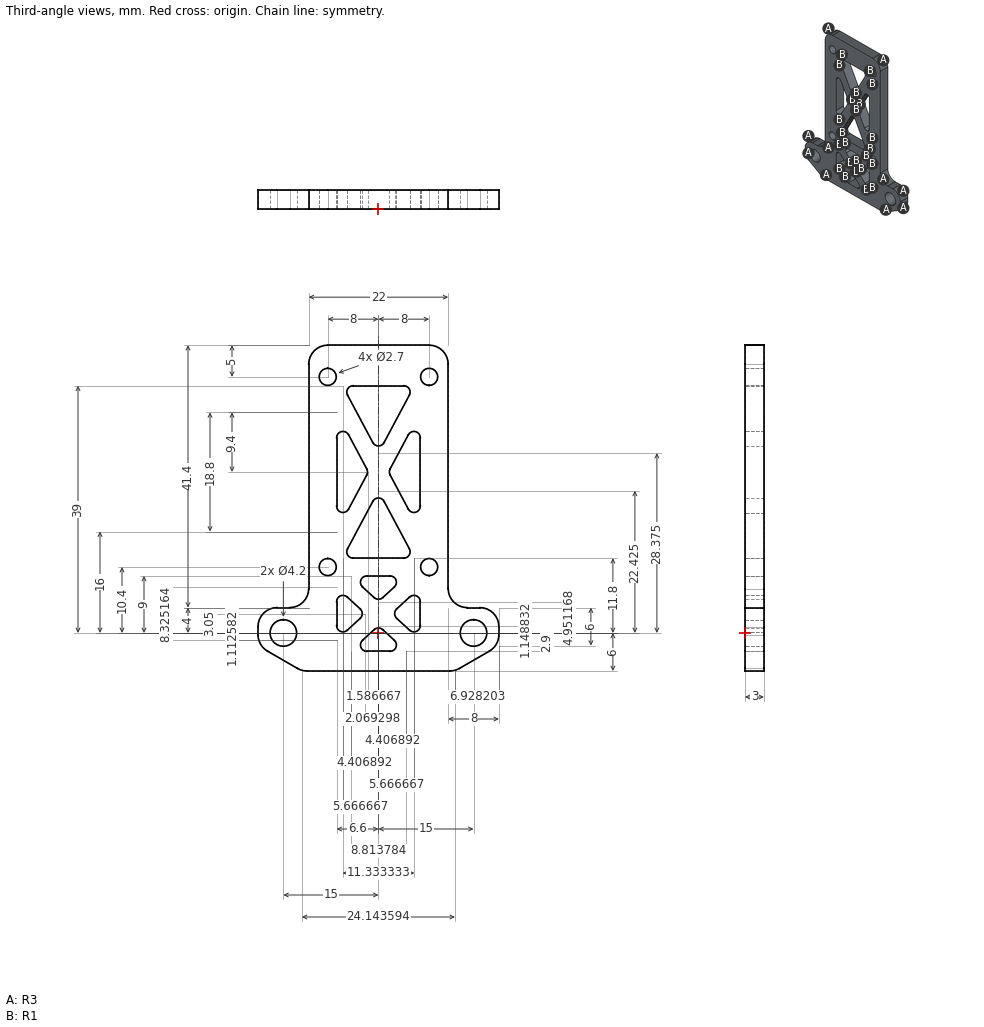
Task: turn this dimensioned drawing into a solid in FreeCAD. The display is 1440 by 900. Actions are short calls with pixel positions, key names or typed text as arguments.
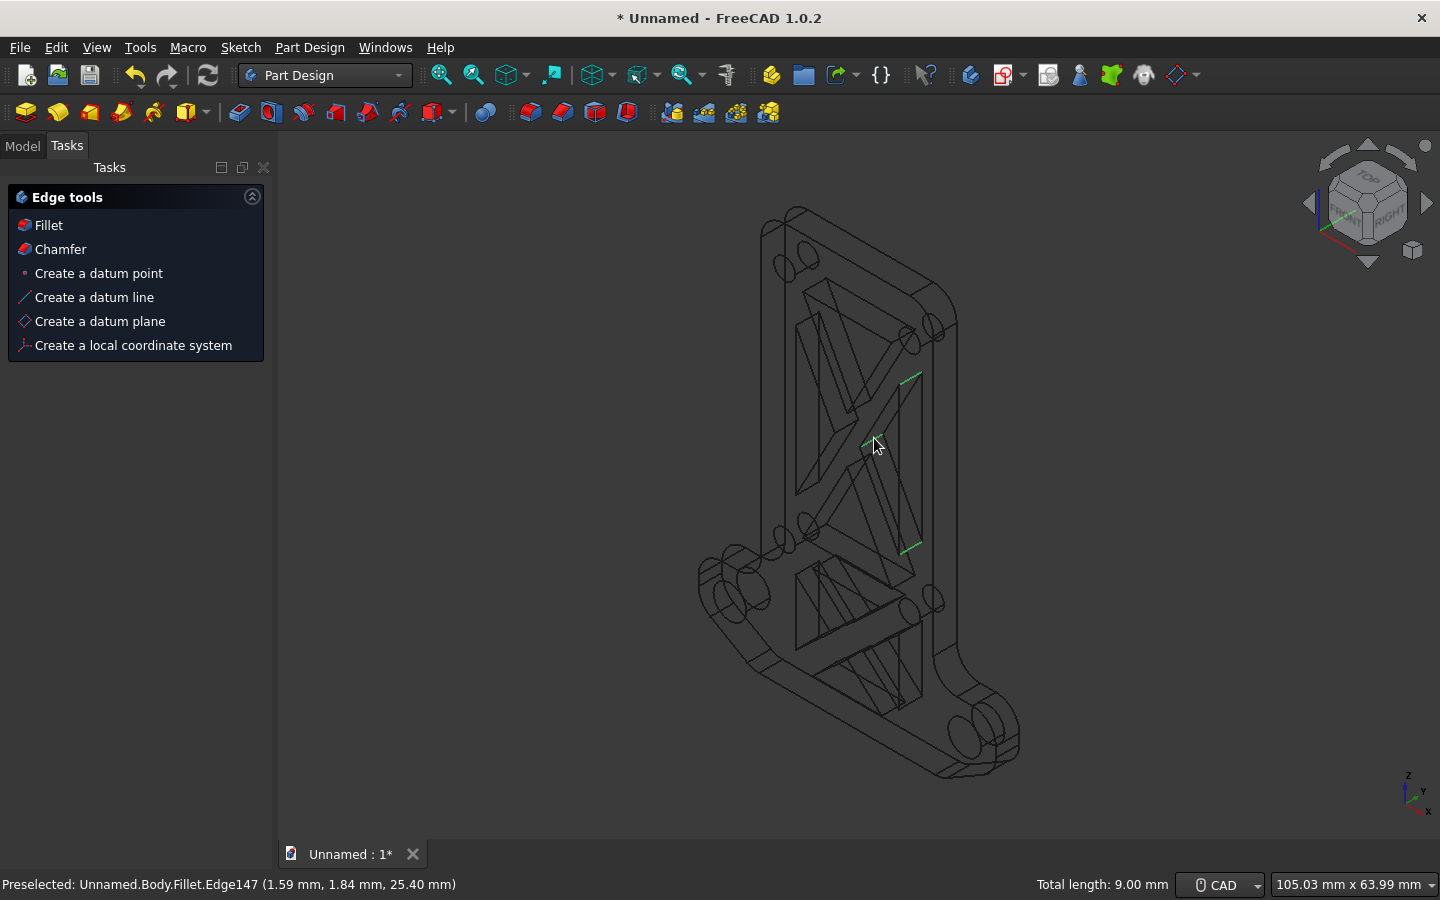
click(805, 319, ctrl)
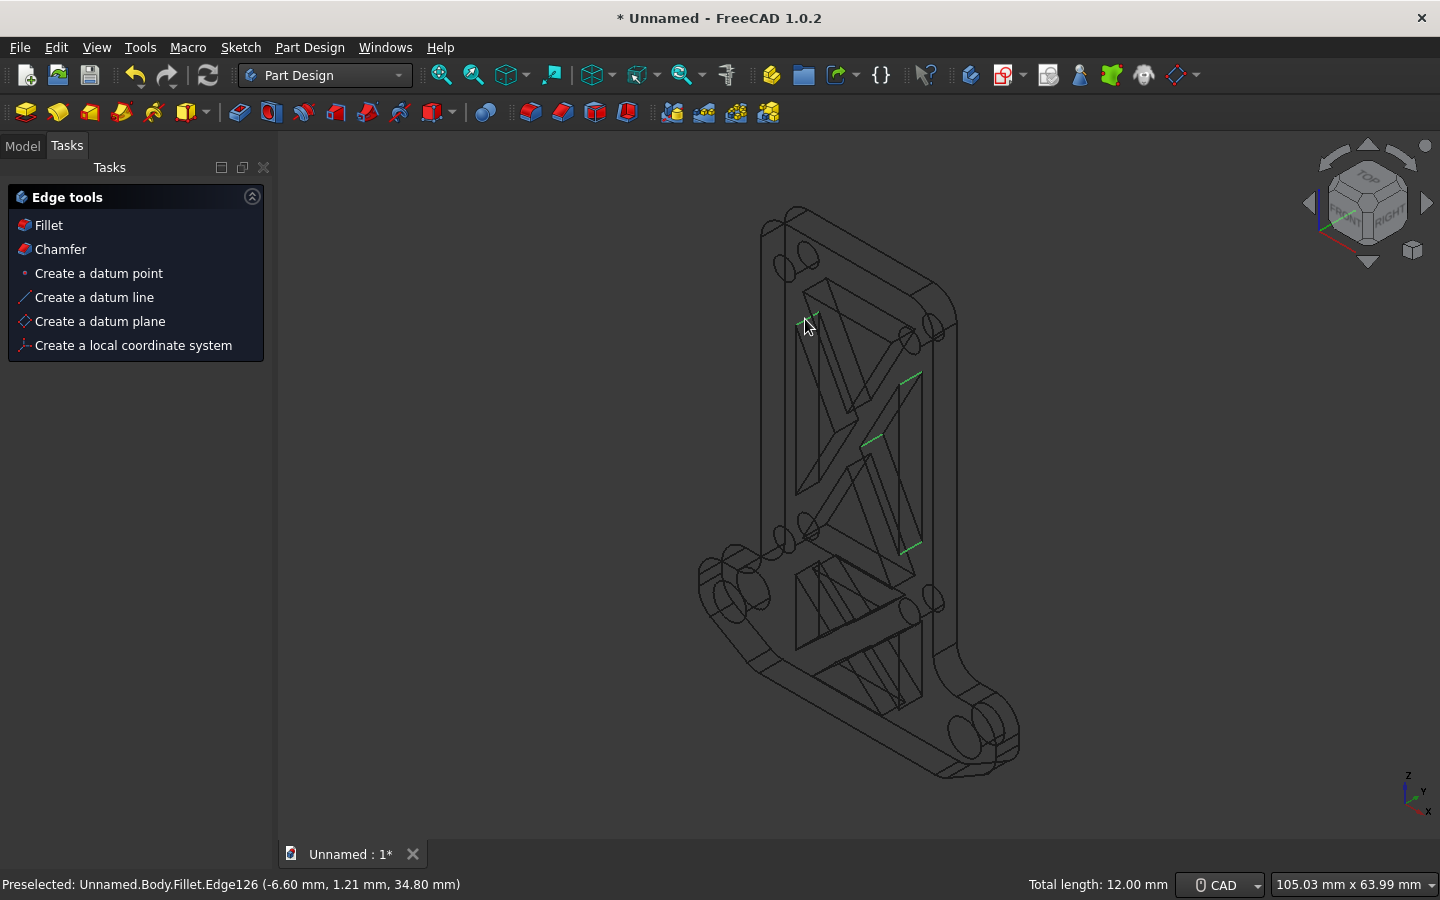
click(810, 486, ctrl)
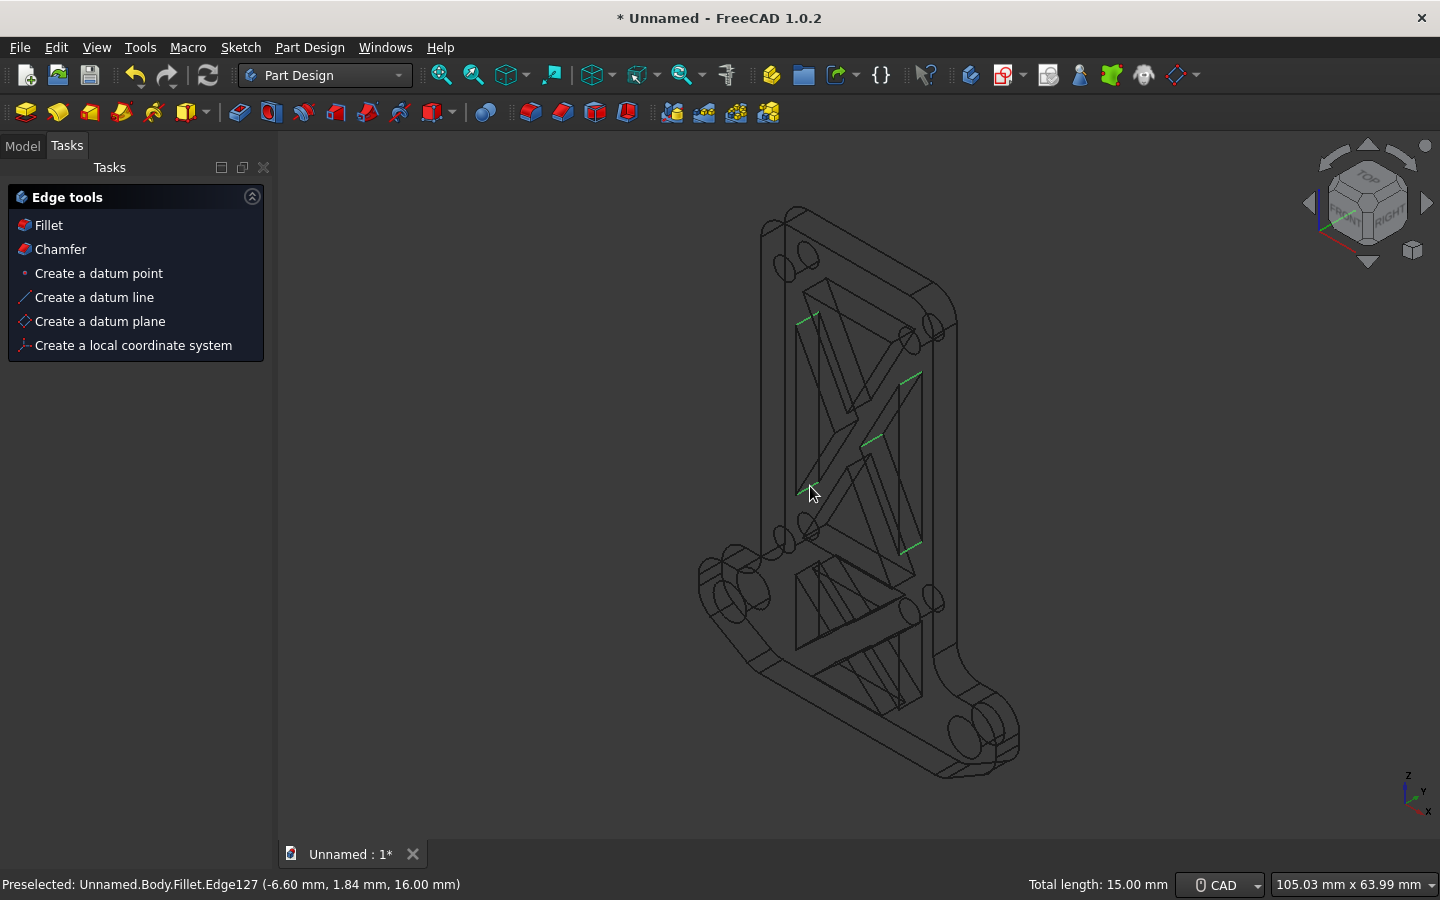
click(847, 425, ctrl)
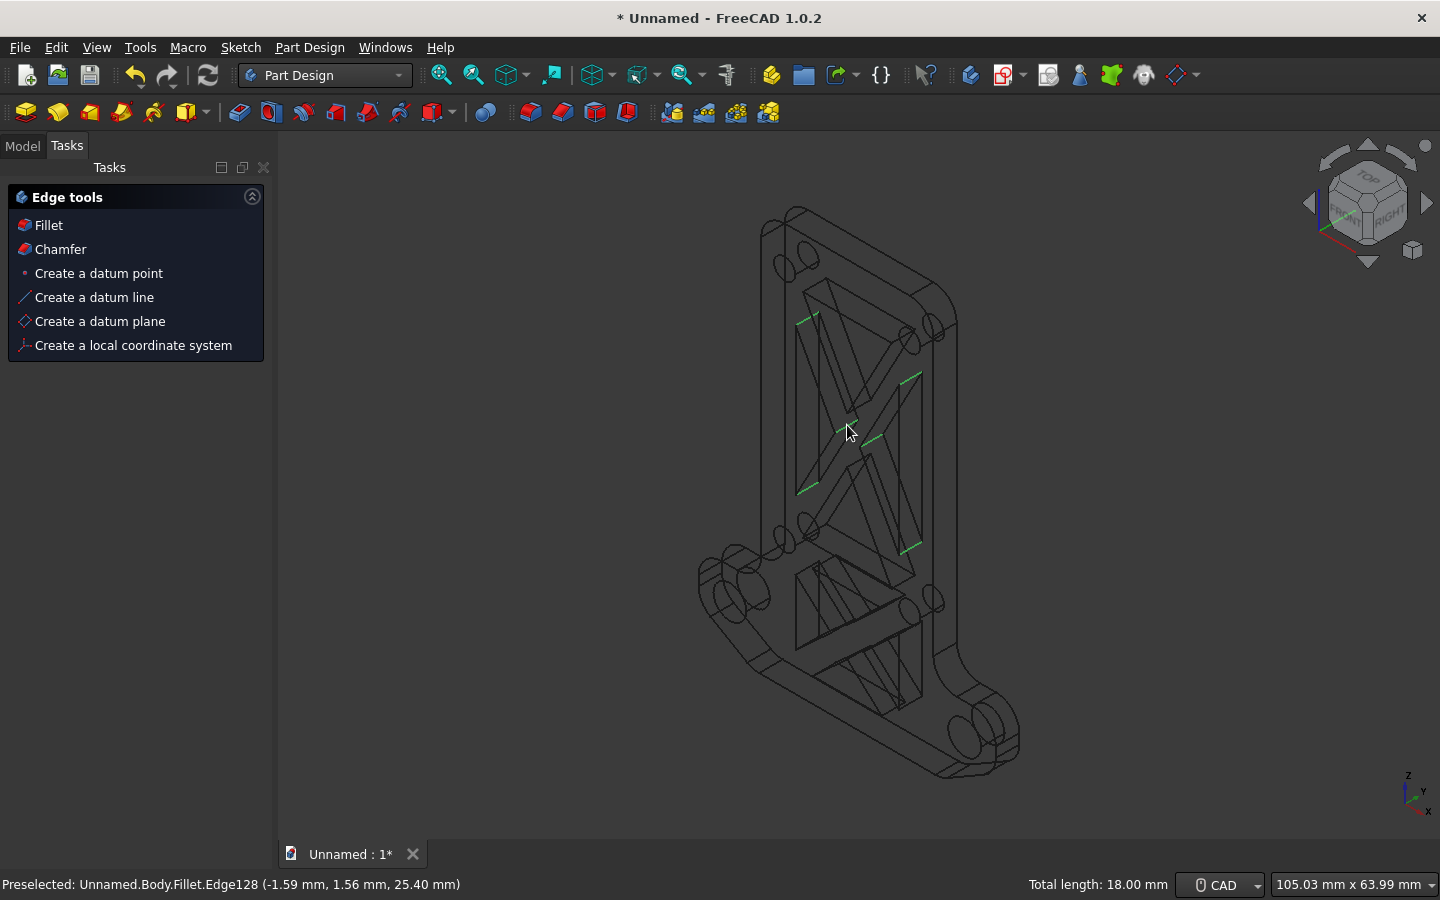
click(906, 334, ctrl)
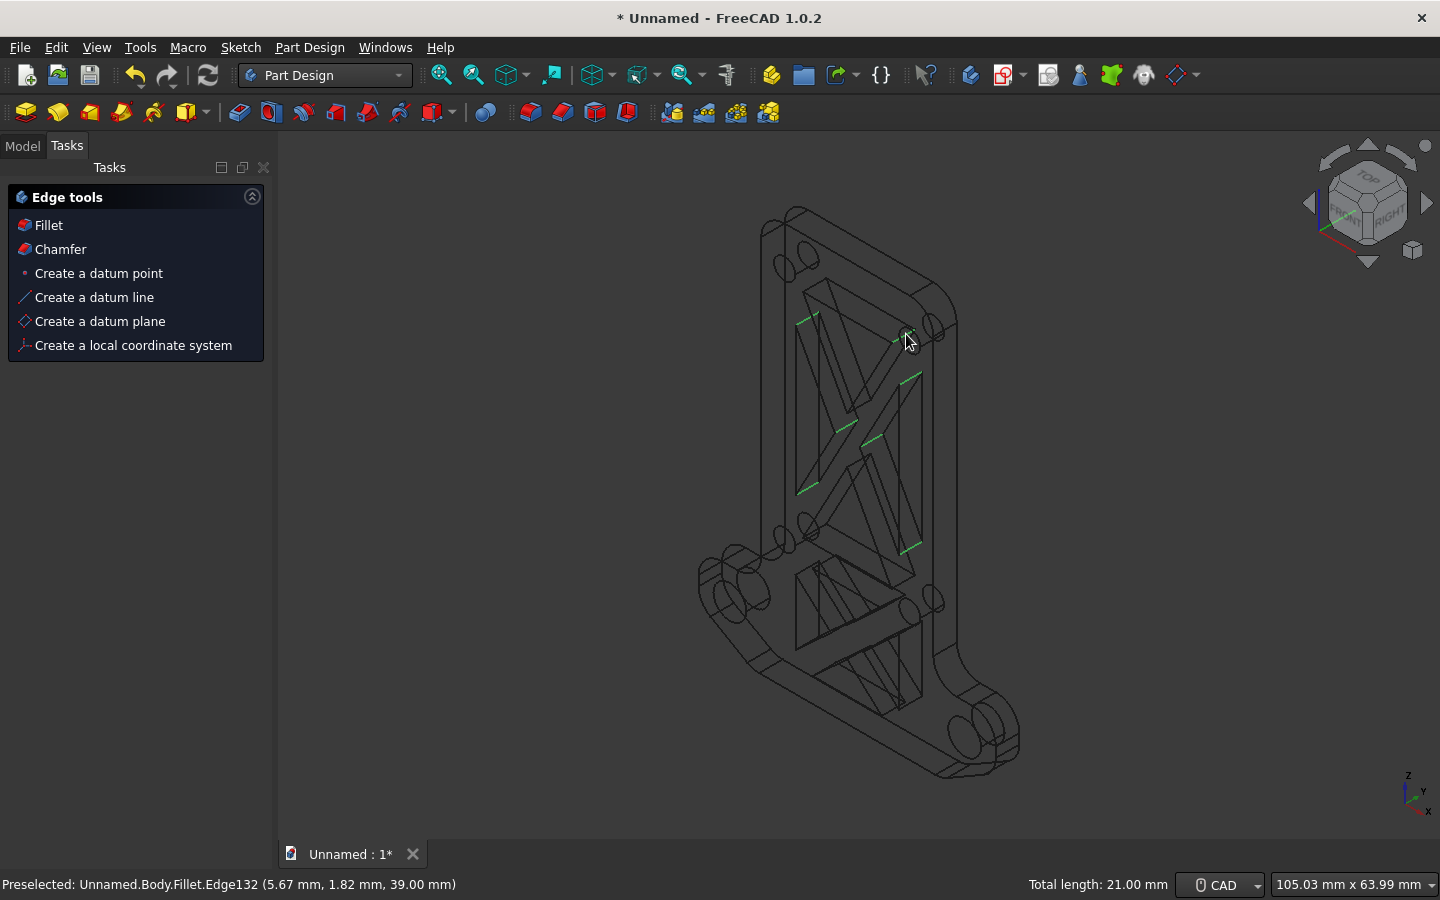
click(815, 284, ctrl)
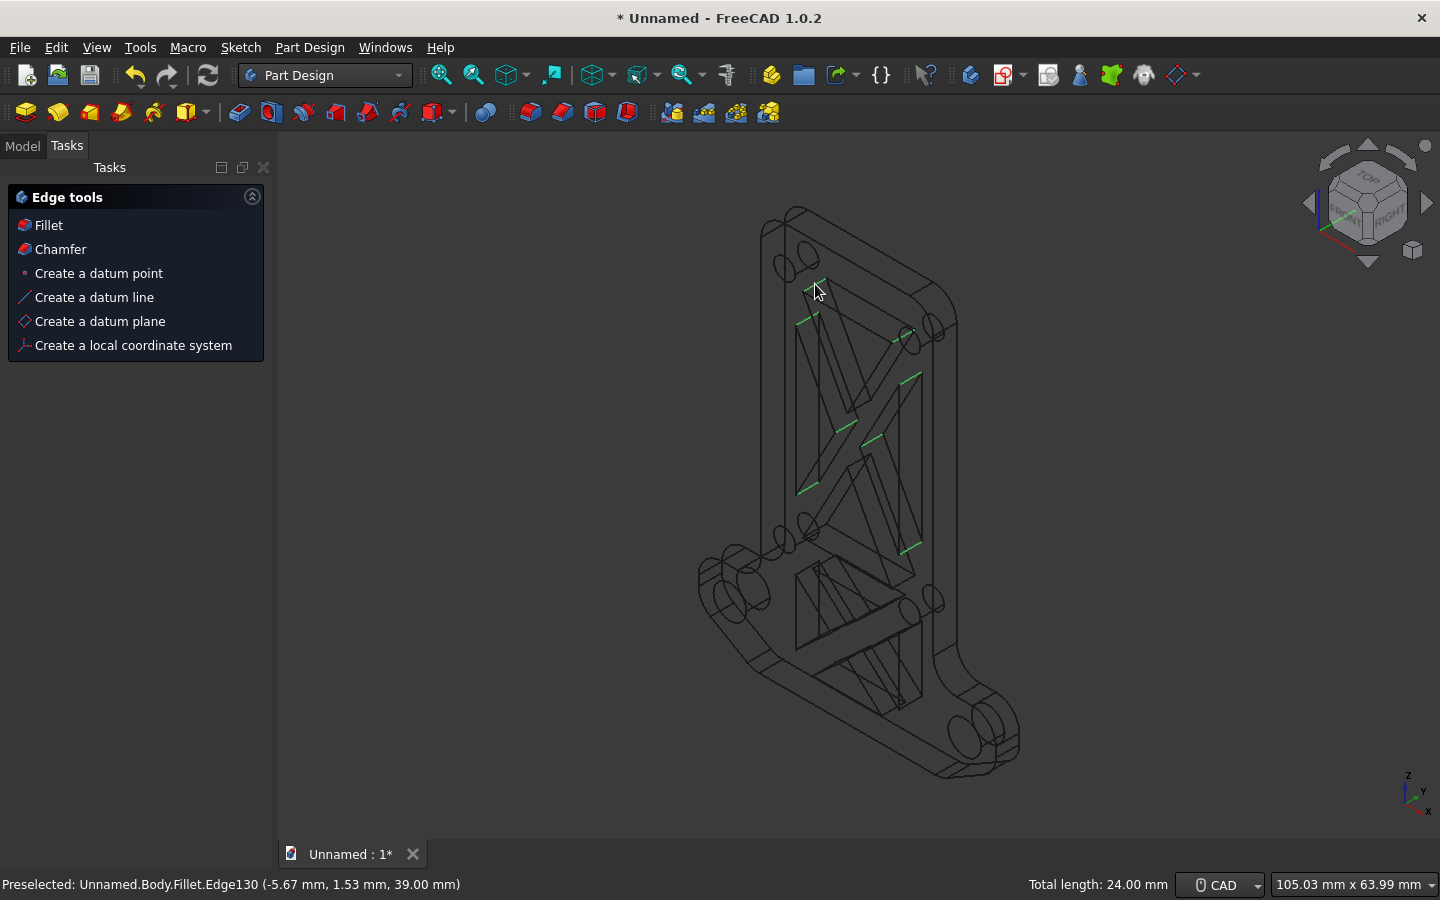
click(859, 406, ctrl)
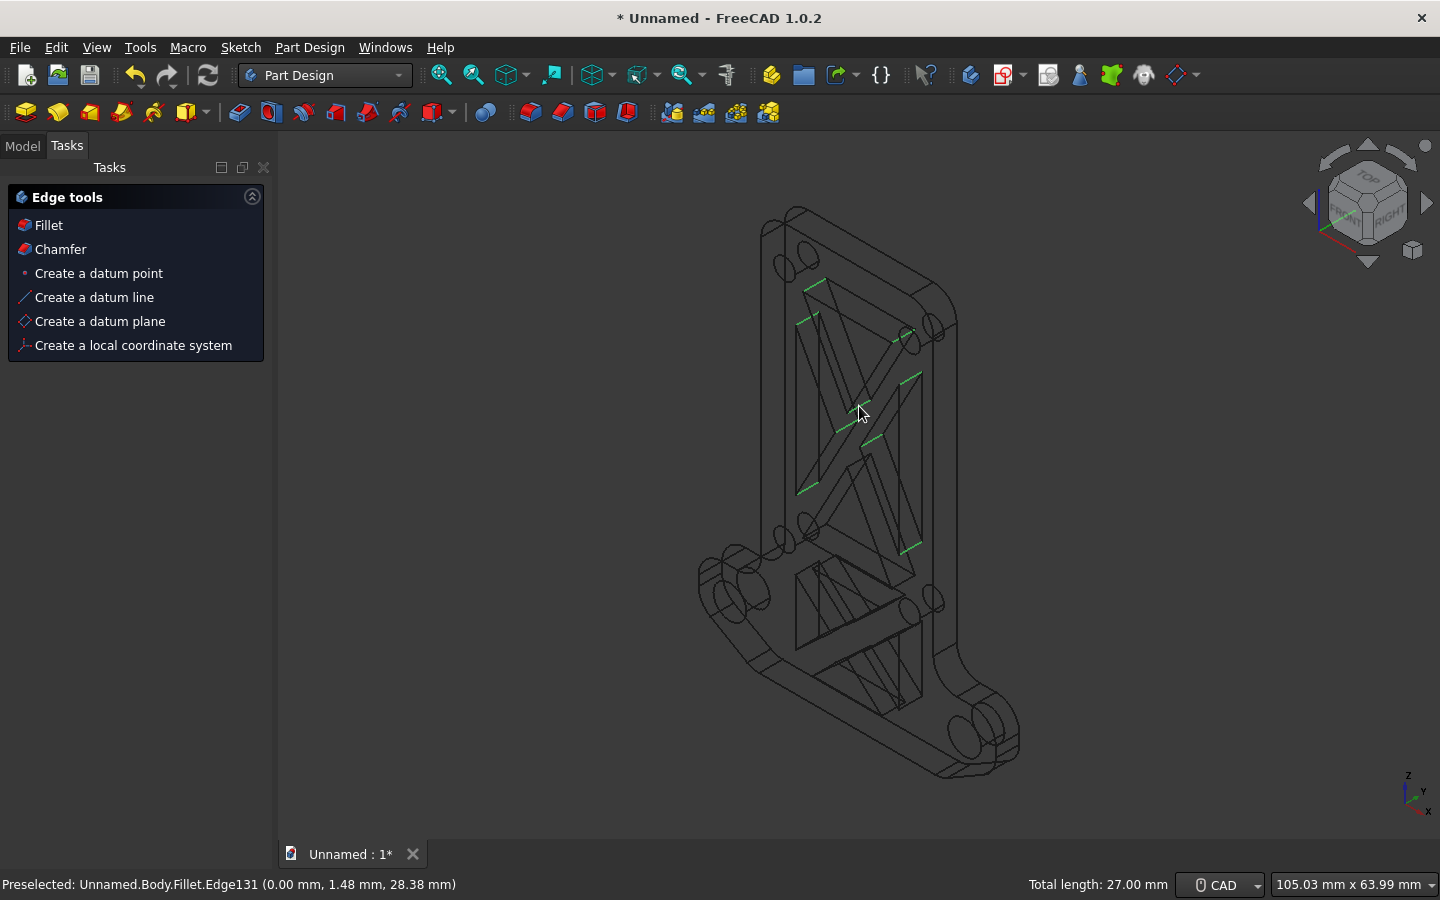
click(840, 626, ctrl)